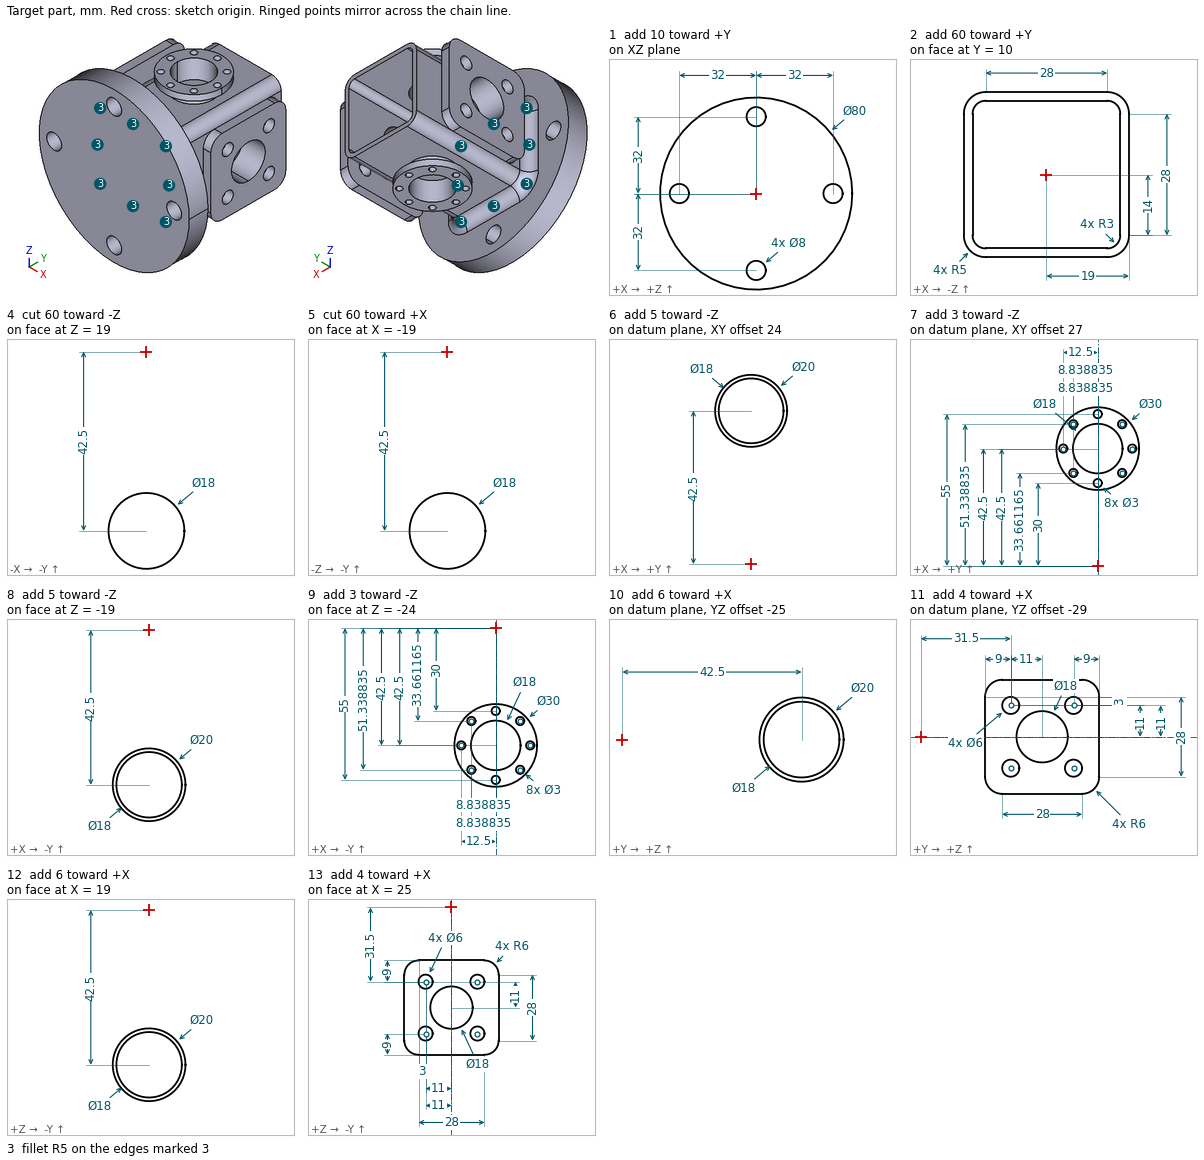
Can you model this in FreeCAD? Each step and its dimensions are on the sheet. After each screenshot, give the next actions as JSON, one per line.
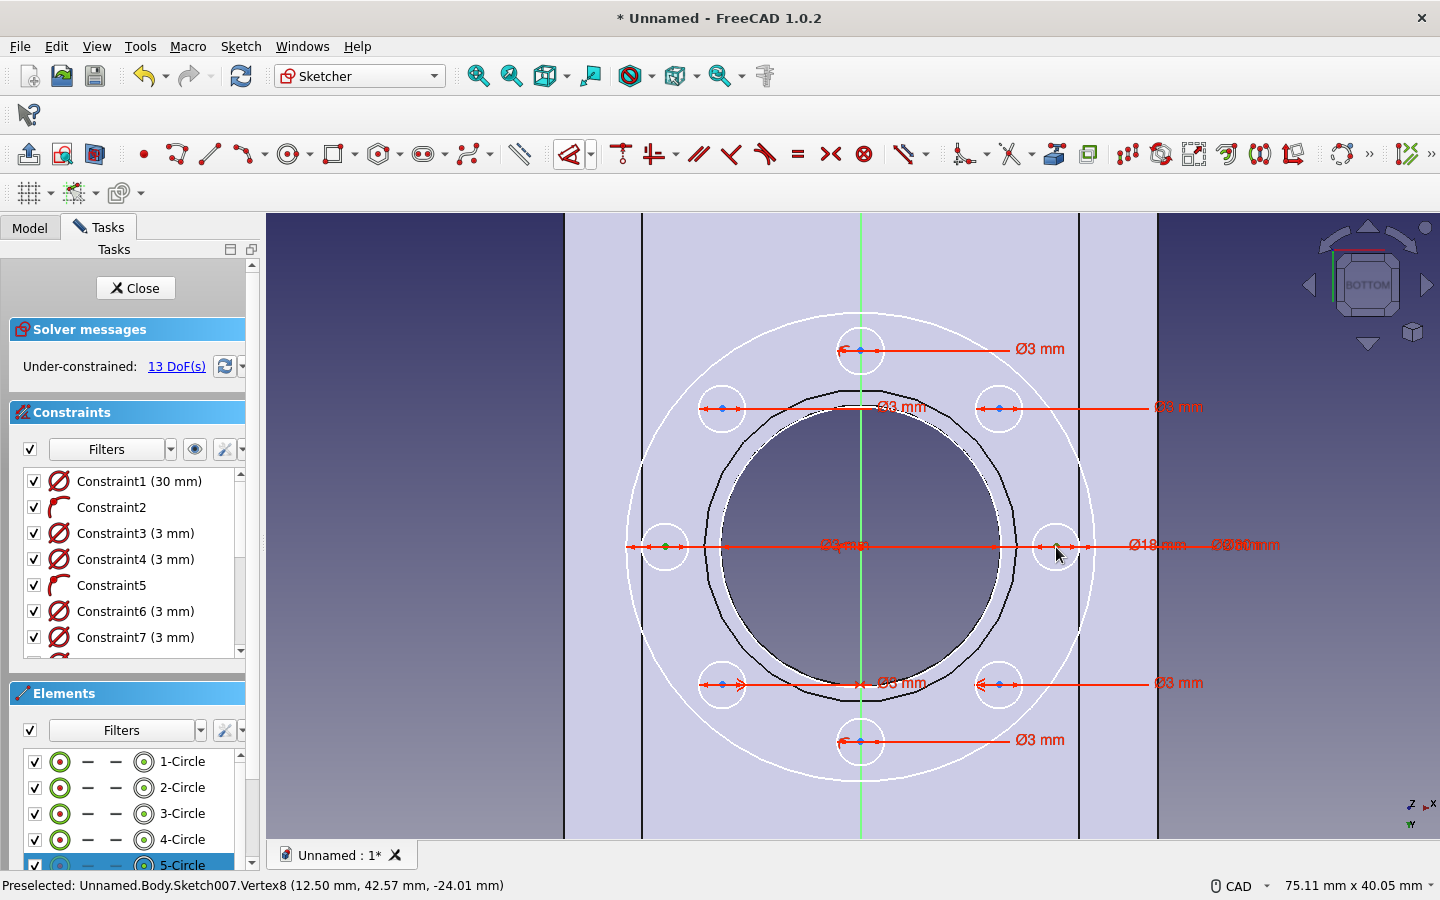
{"action": "left_click", "coordinate": [861, 648]}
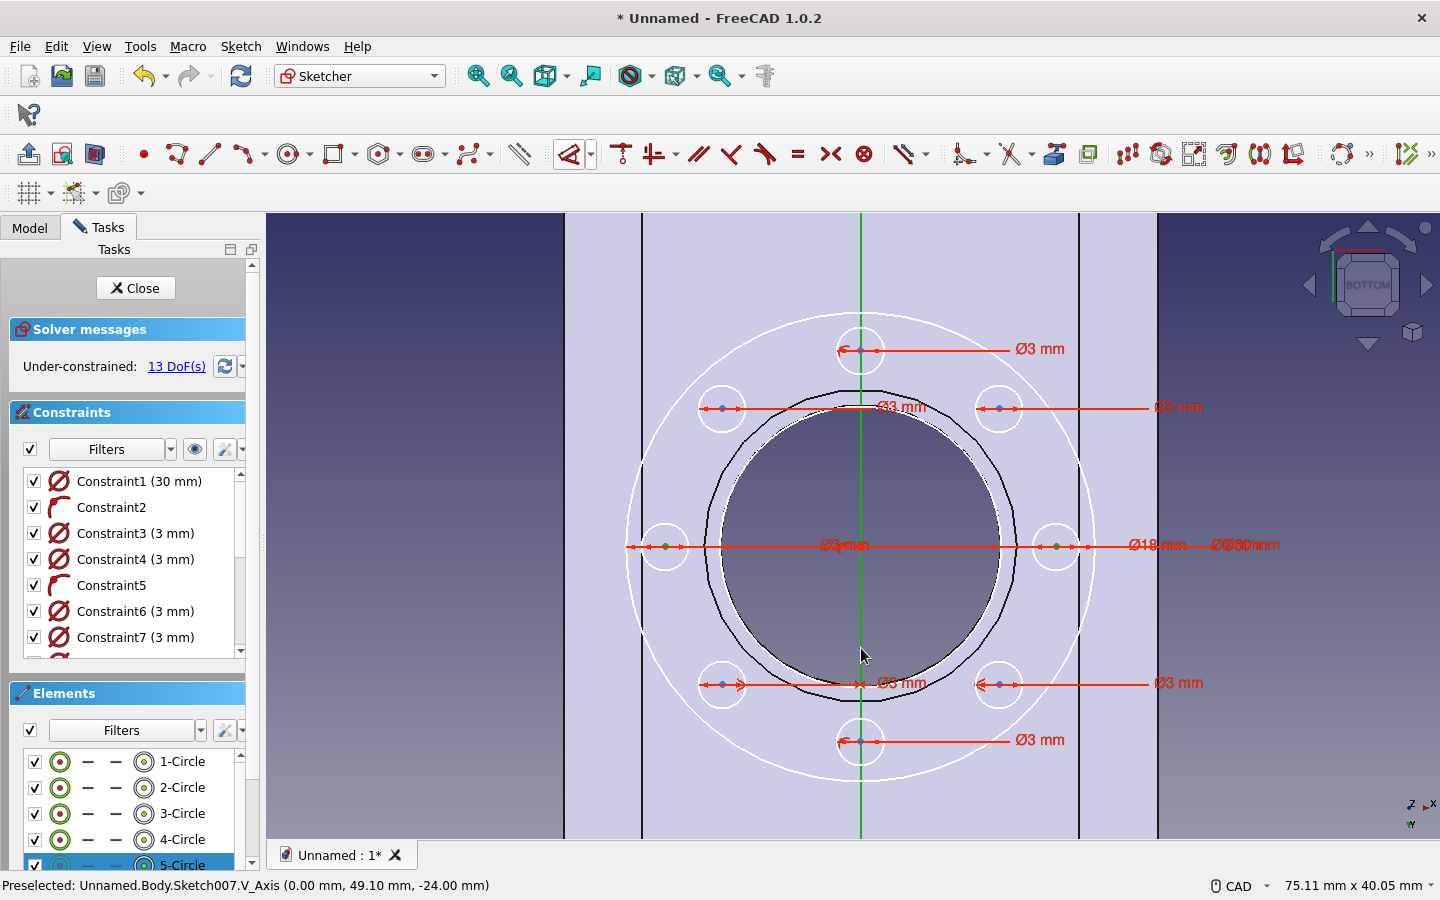
{"action": "key", "text": "s"}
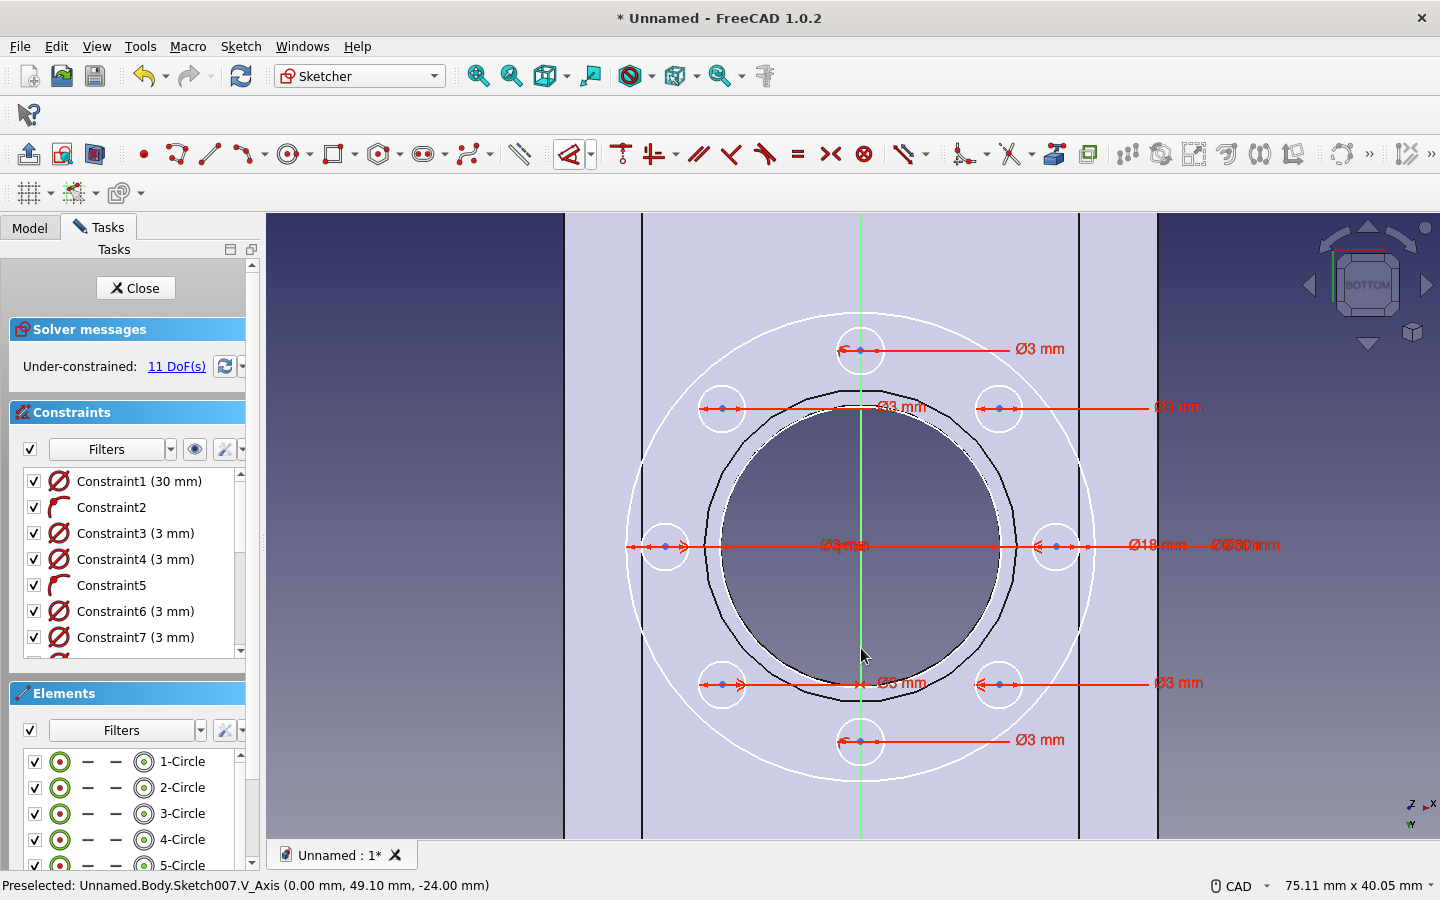
{"action": "left_click", "coordinate": [722, 409]}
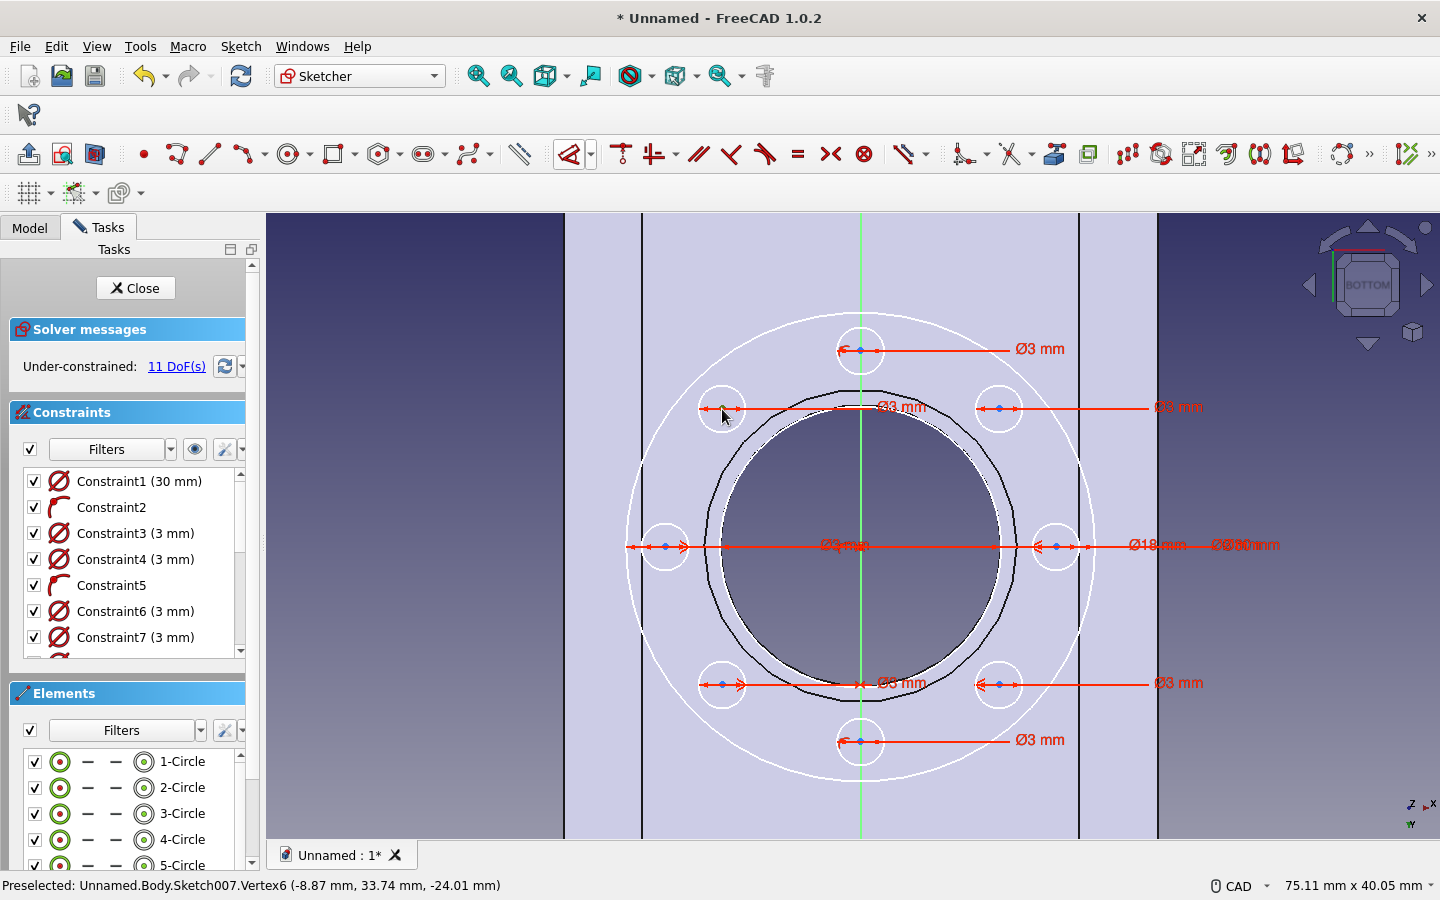
{"action": "left_click", "coordinate": [999, 409]}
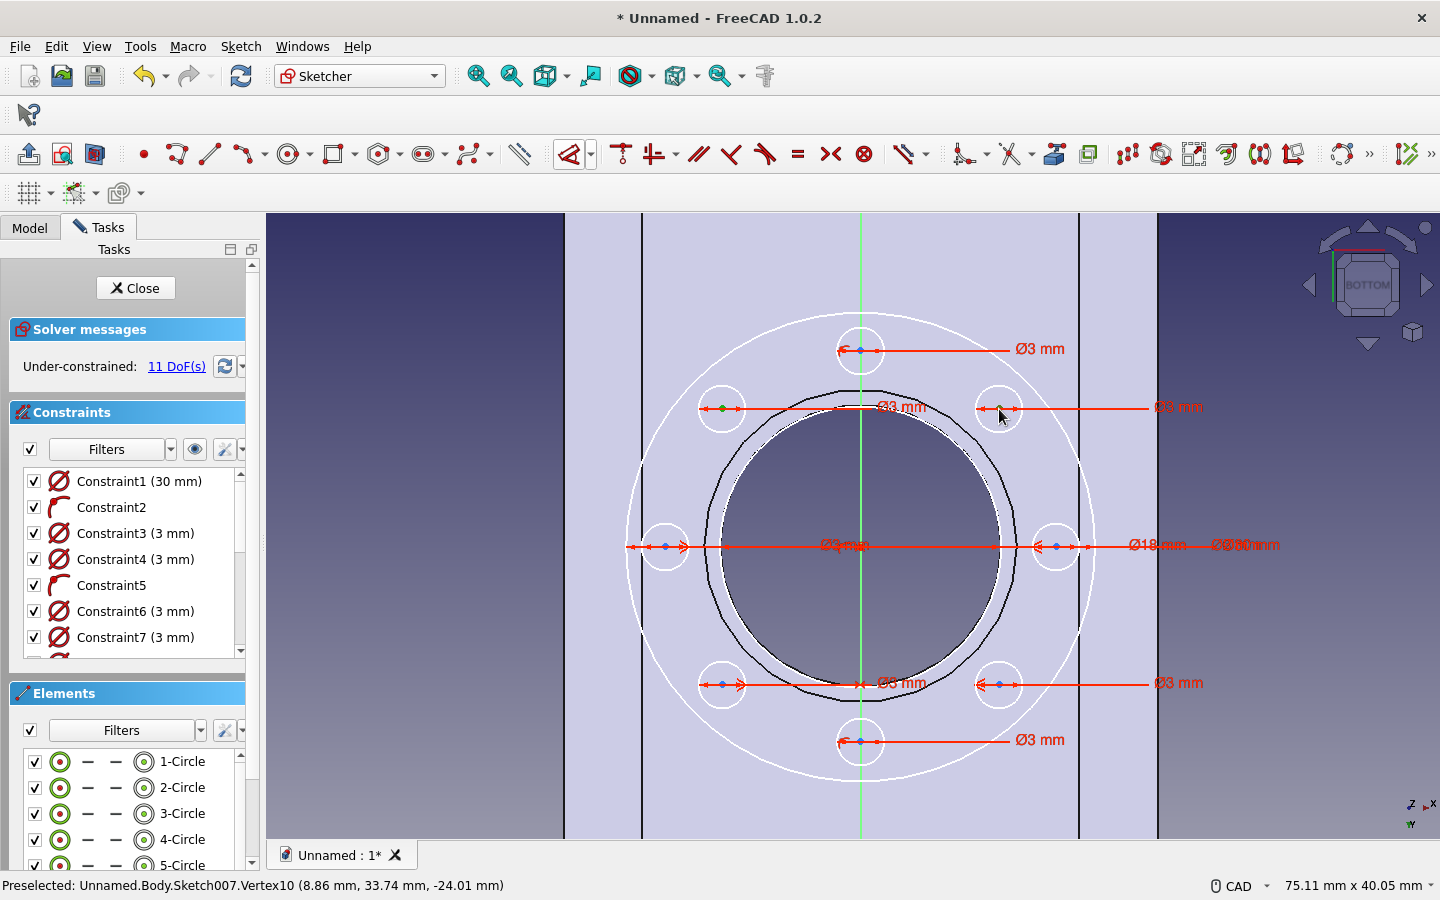
{"action": "left_click", "coordinate": [861, 648]}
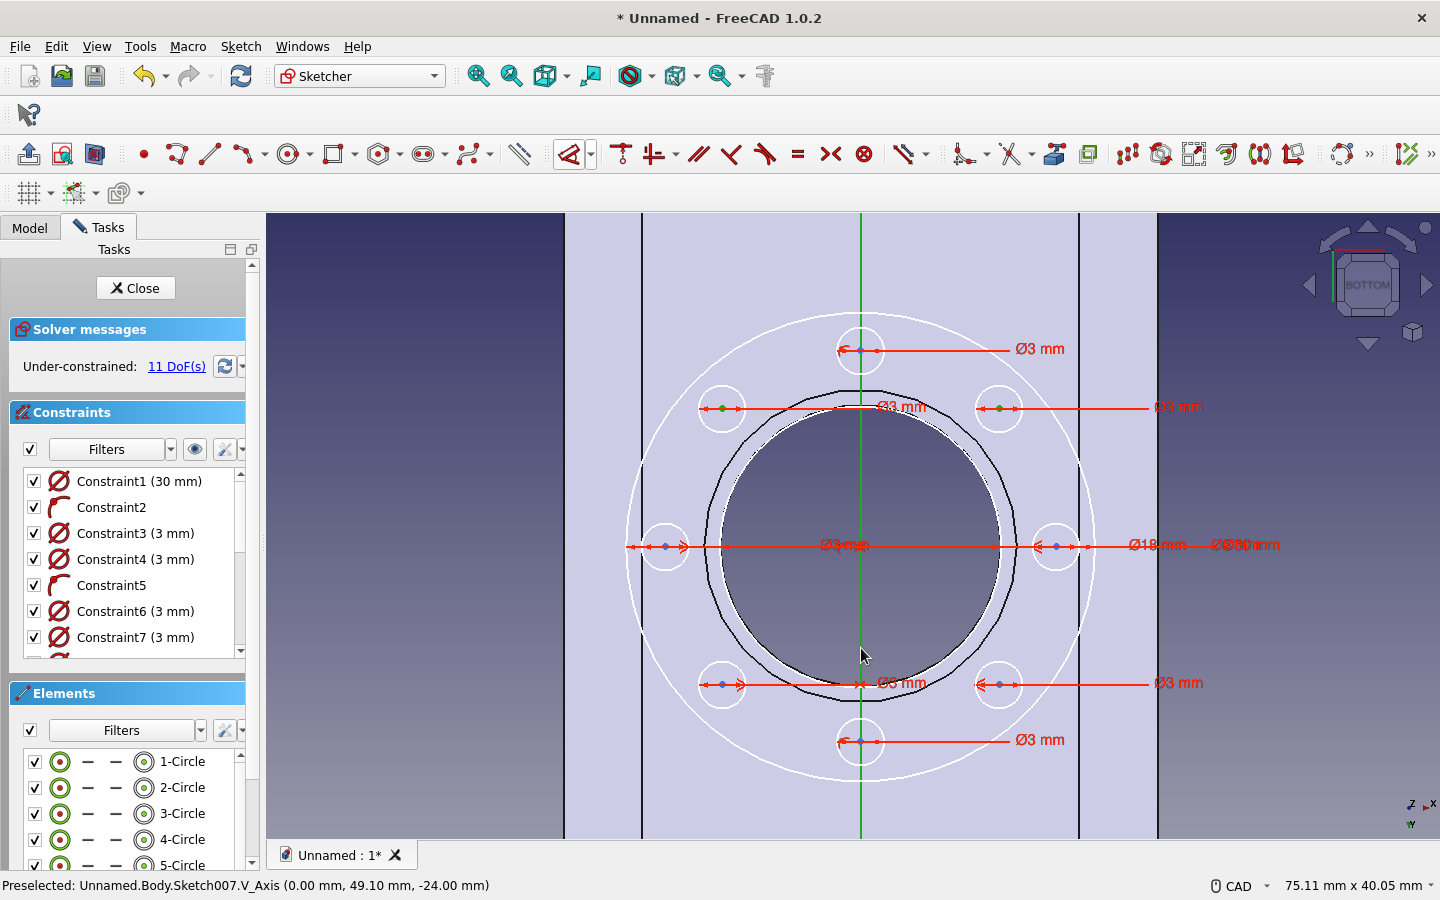
{"action": "left_click", "coordinate": [831, 154]}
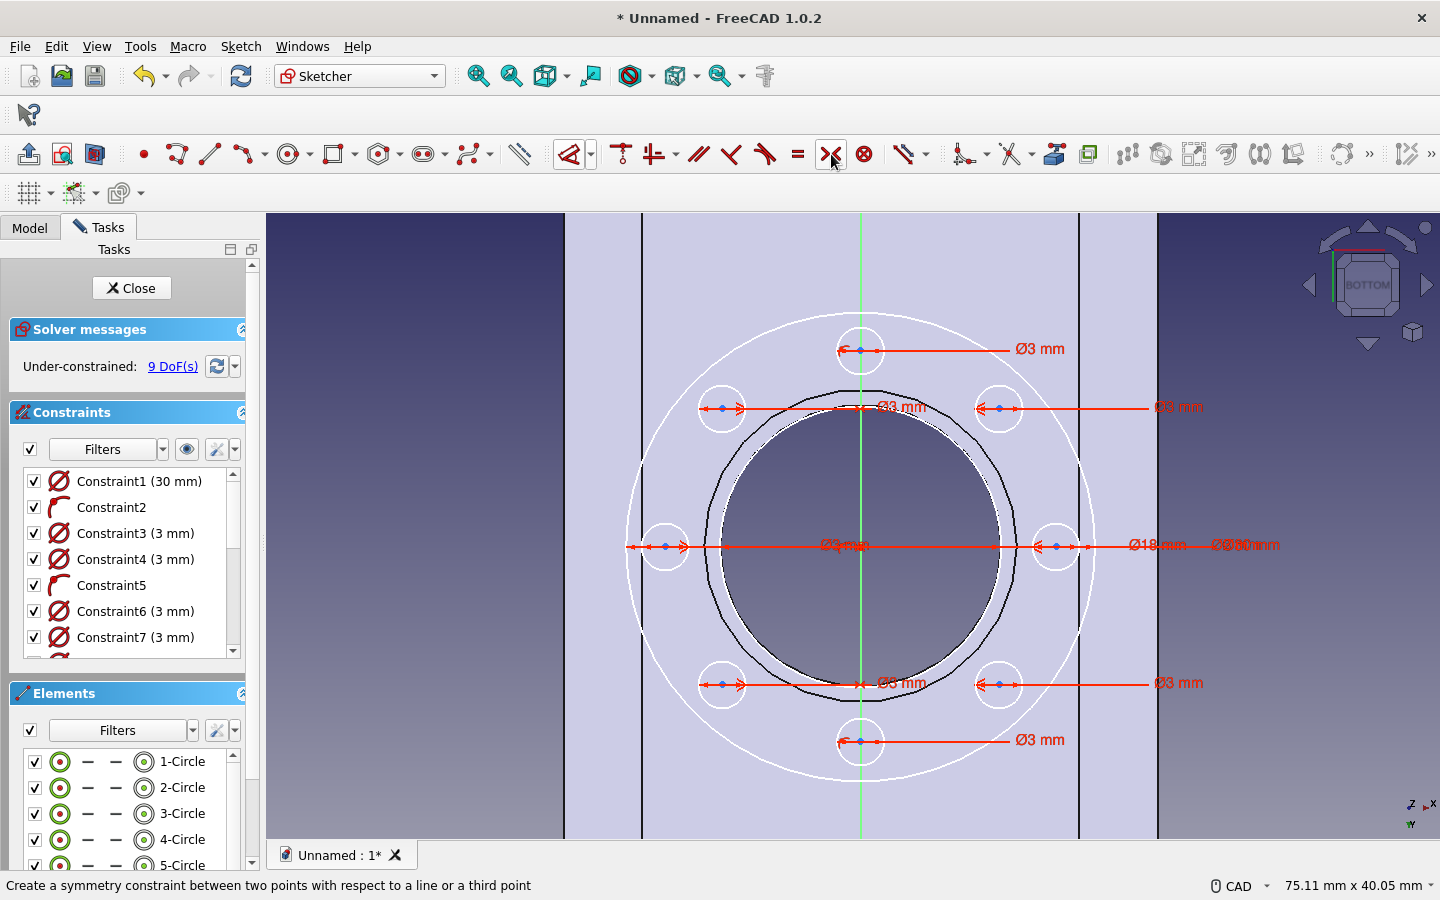
{"action": "left_click", "coordinate": [861, 742]}